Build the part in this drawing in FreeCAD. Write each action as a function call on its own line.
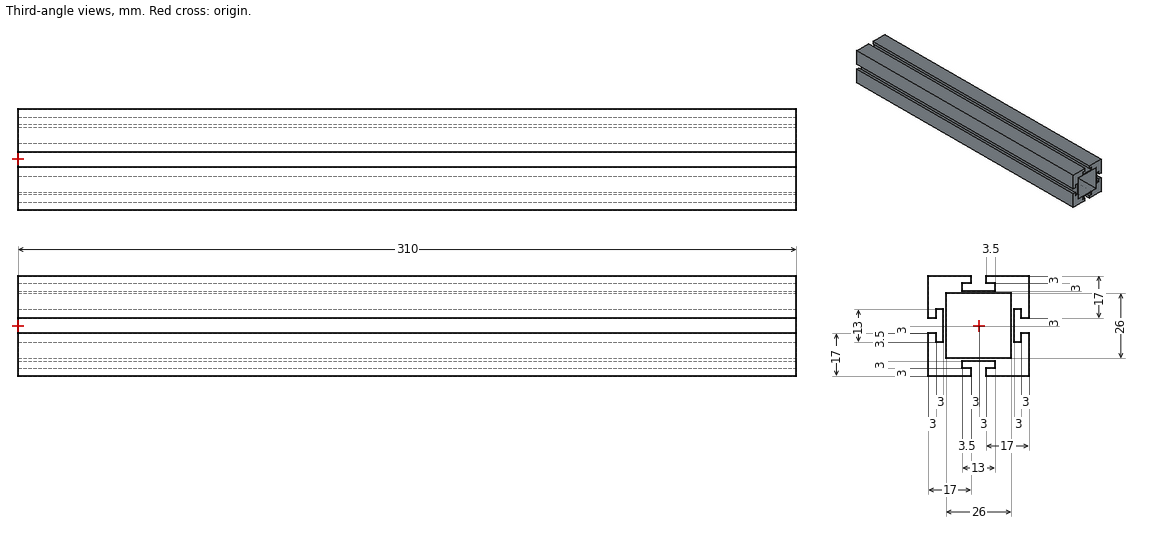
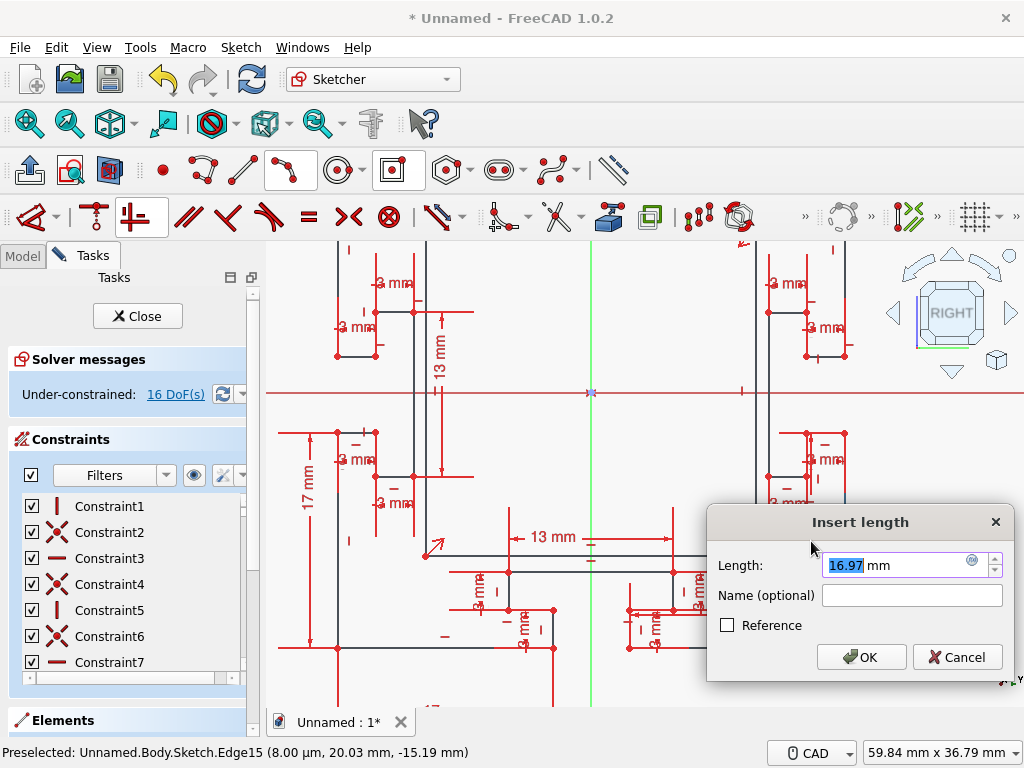
text(17)
key(Return)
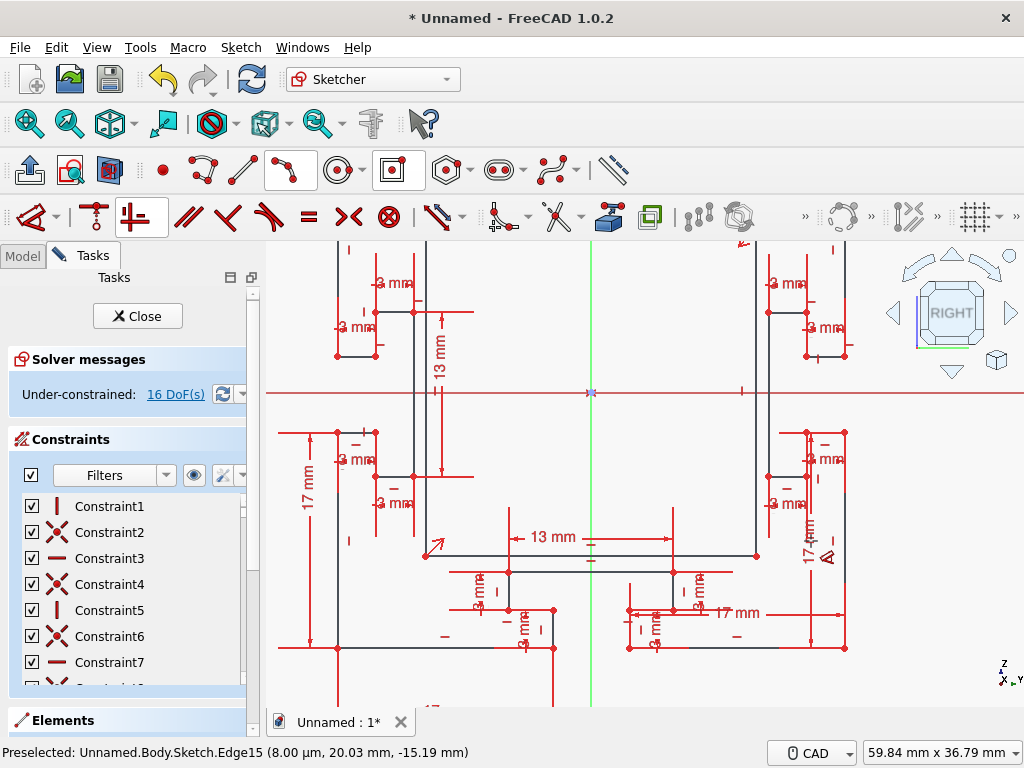
click(769, 428)
click(735, 357)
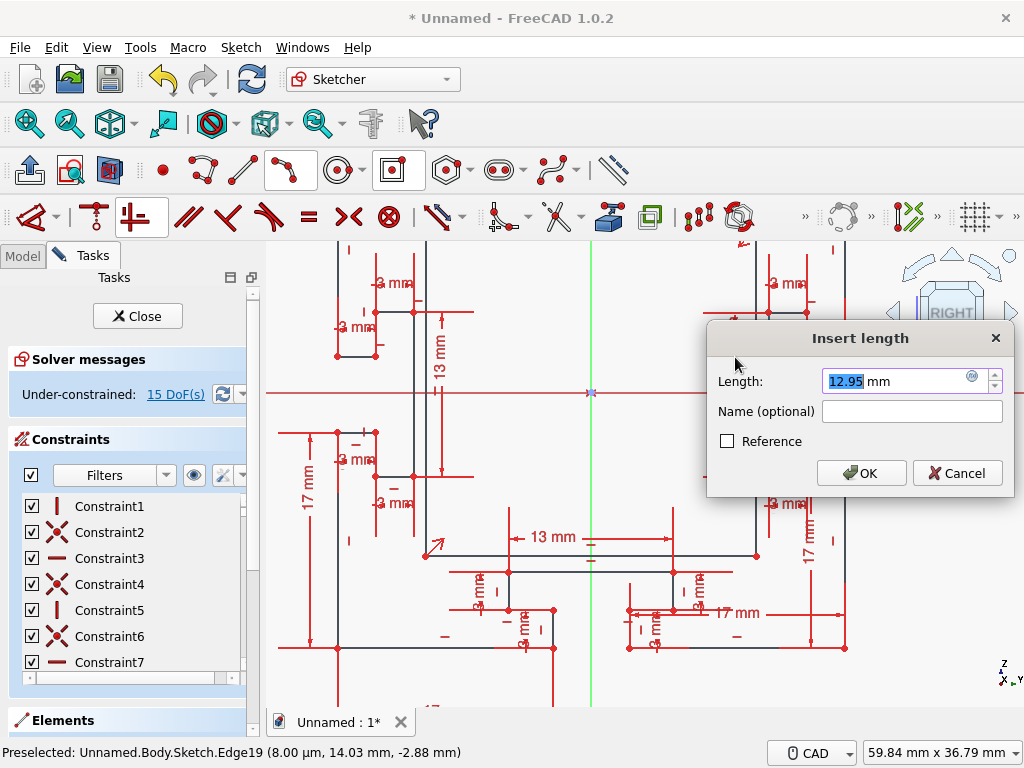
text(13)
key(Return)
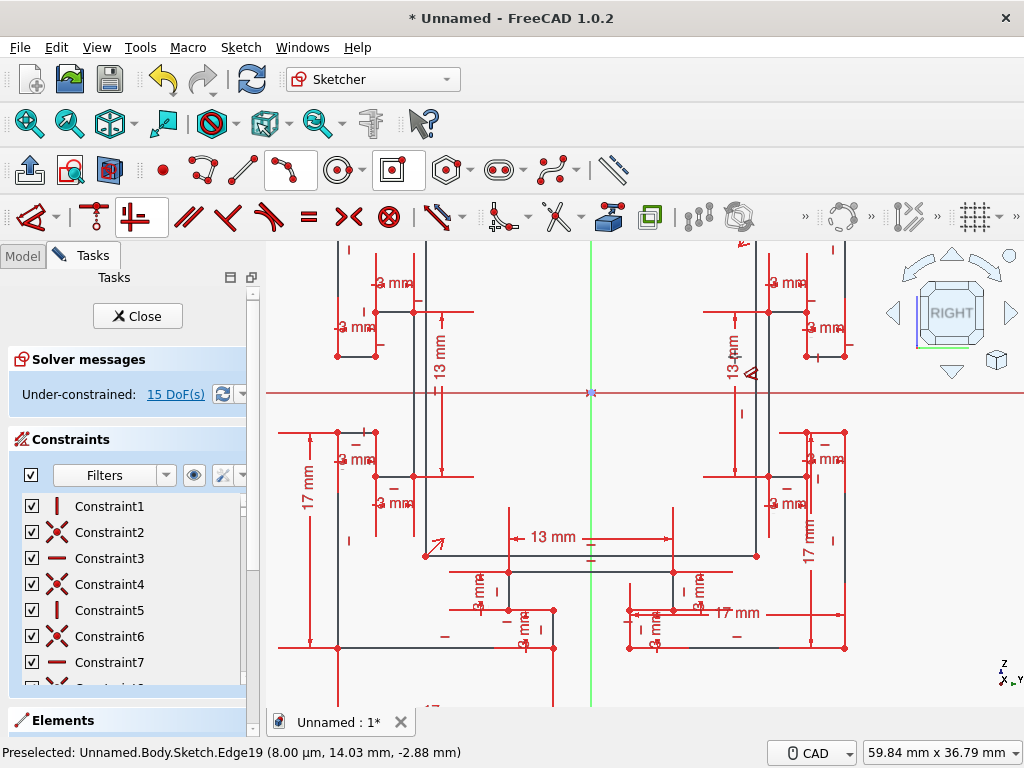
click(845, 292)
click(739, 313)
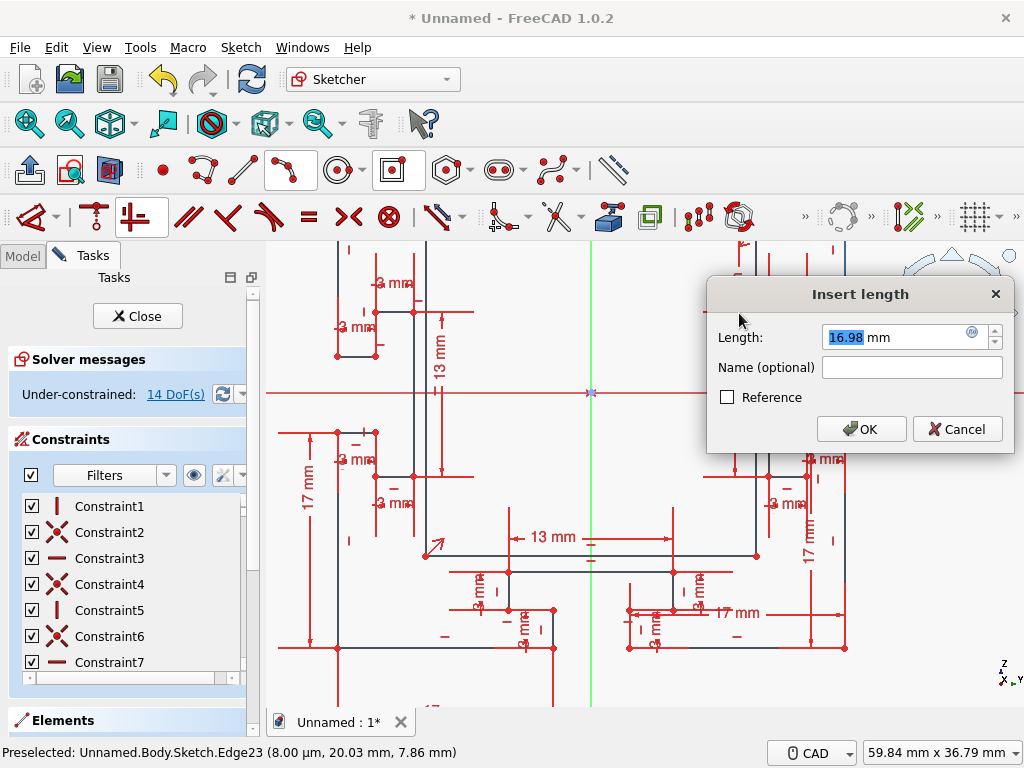
text(17)
key(Return)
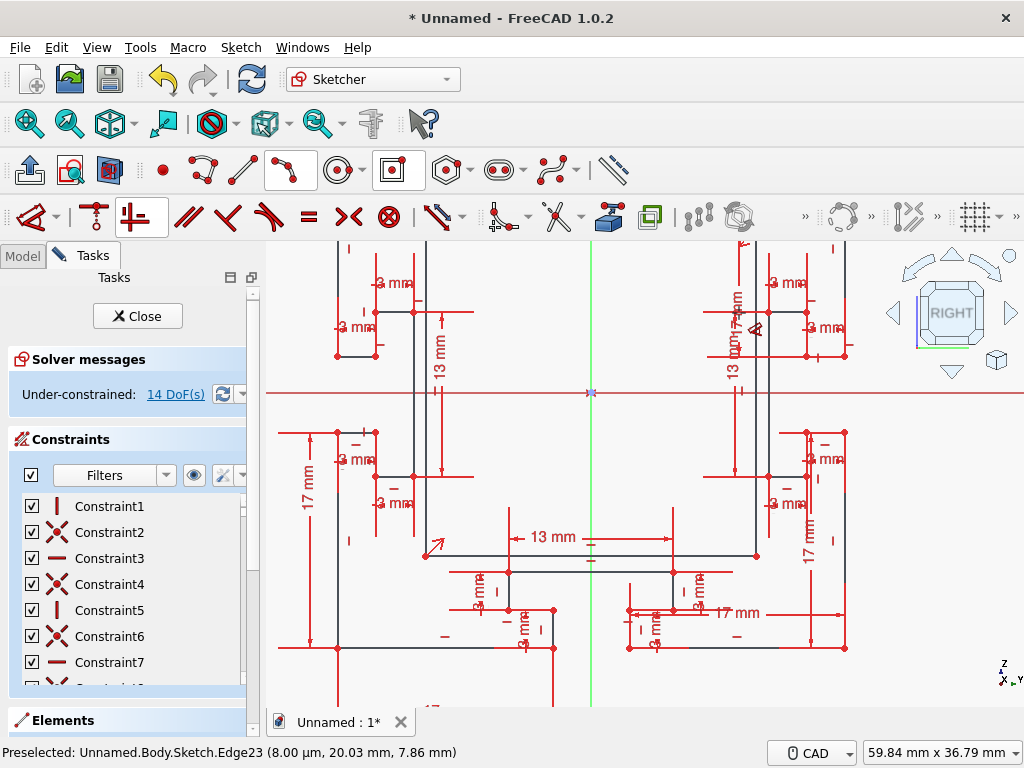
scroll(559, 573, down, 3)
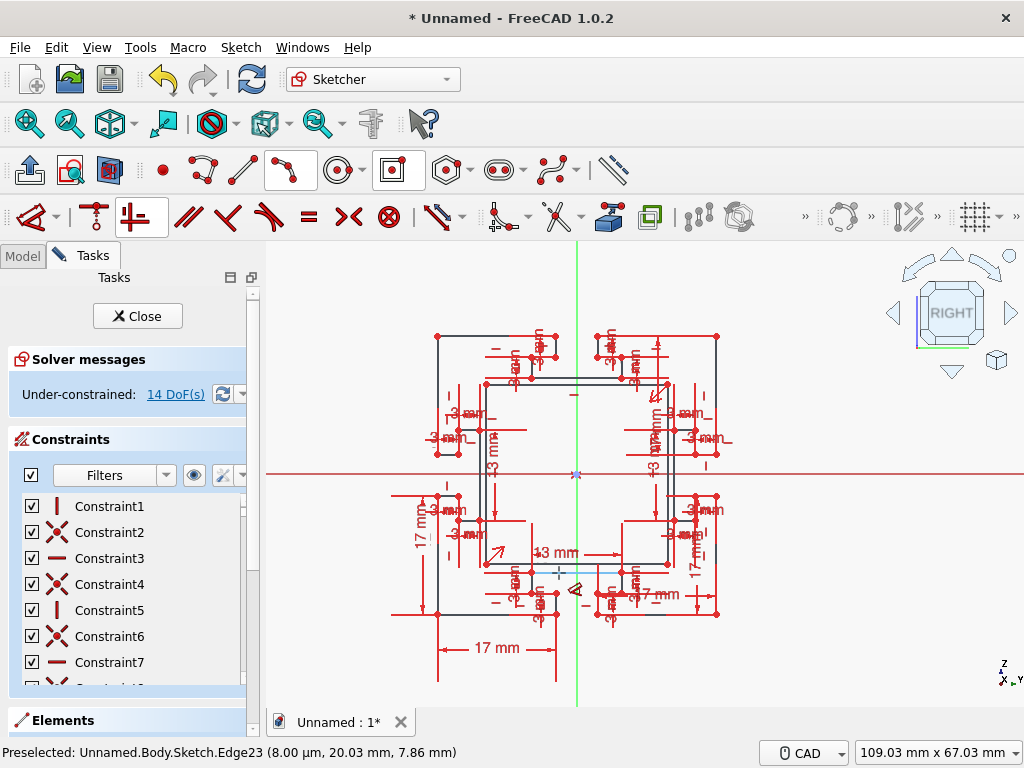
click(681, 336)
click(657, 302)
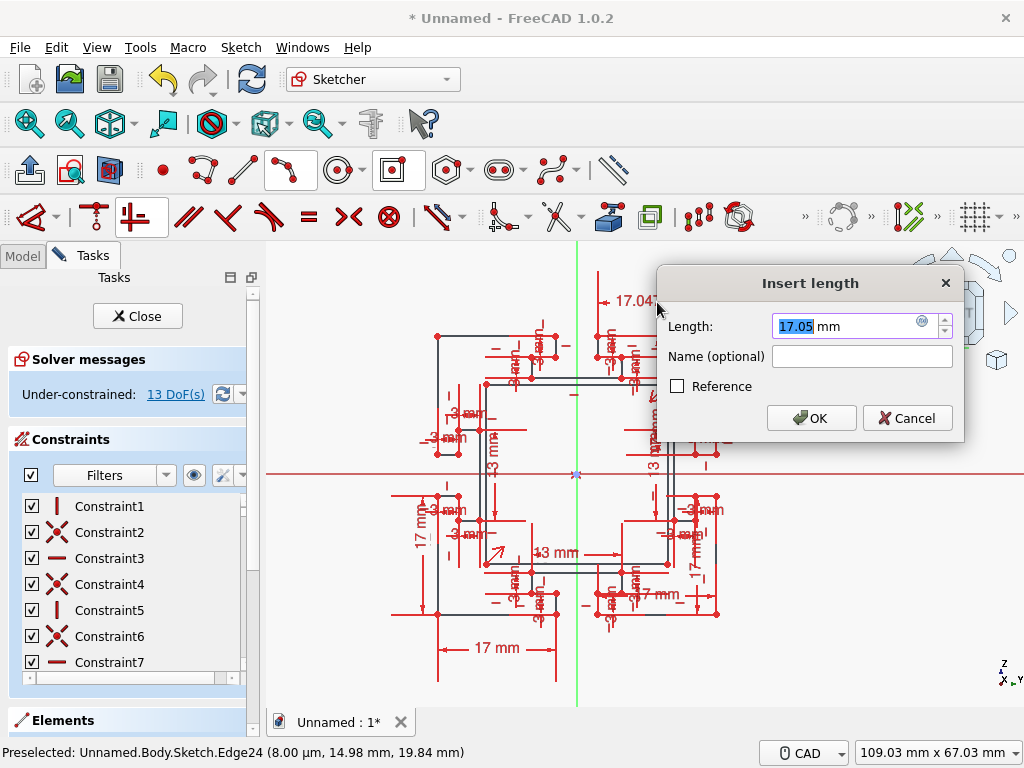
text(17)
key(Return)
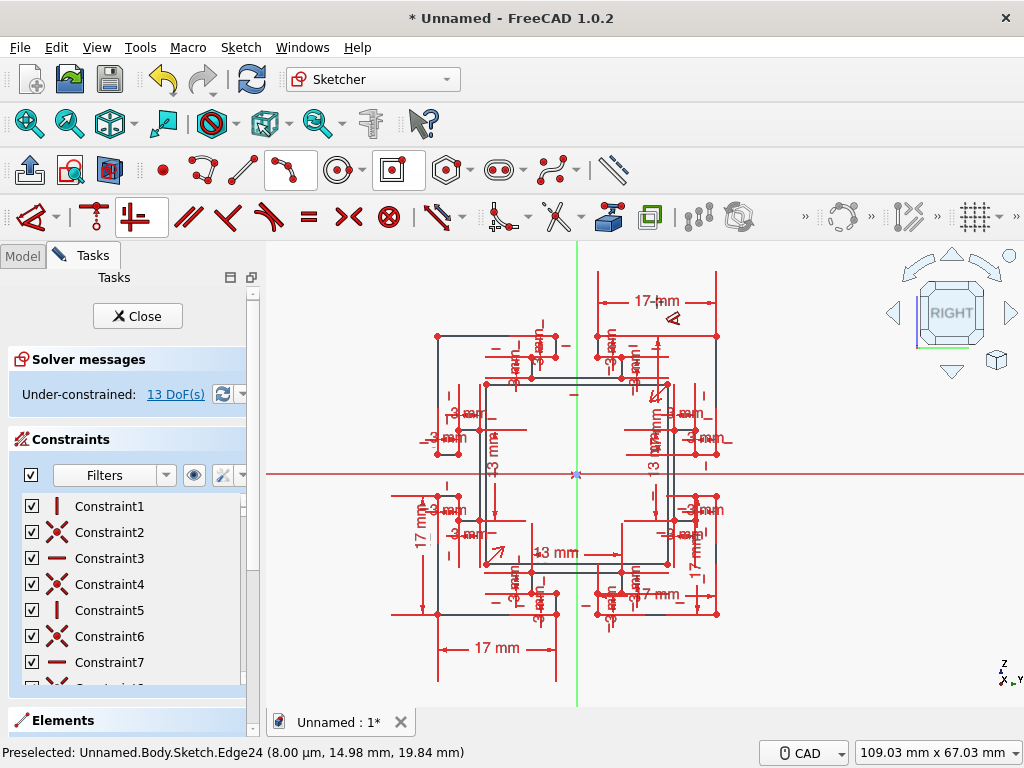
scroll(595, 378, up, 4)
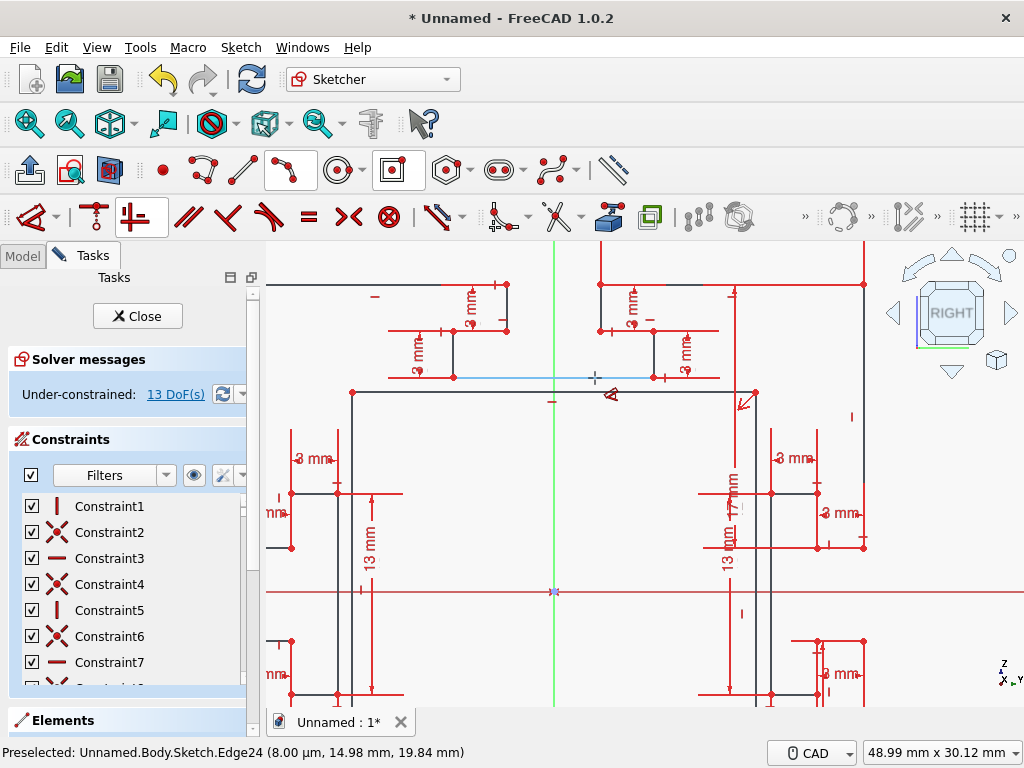
click(593, 378)
click(507, 412)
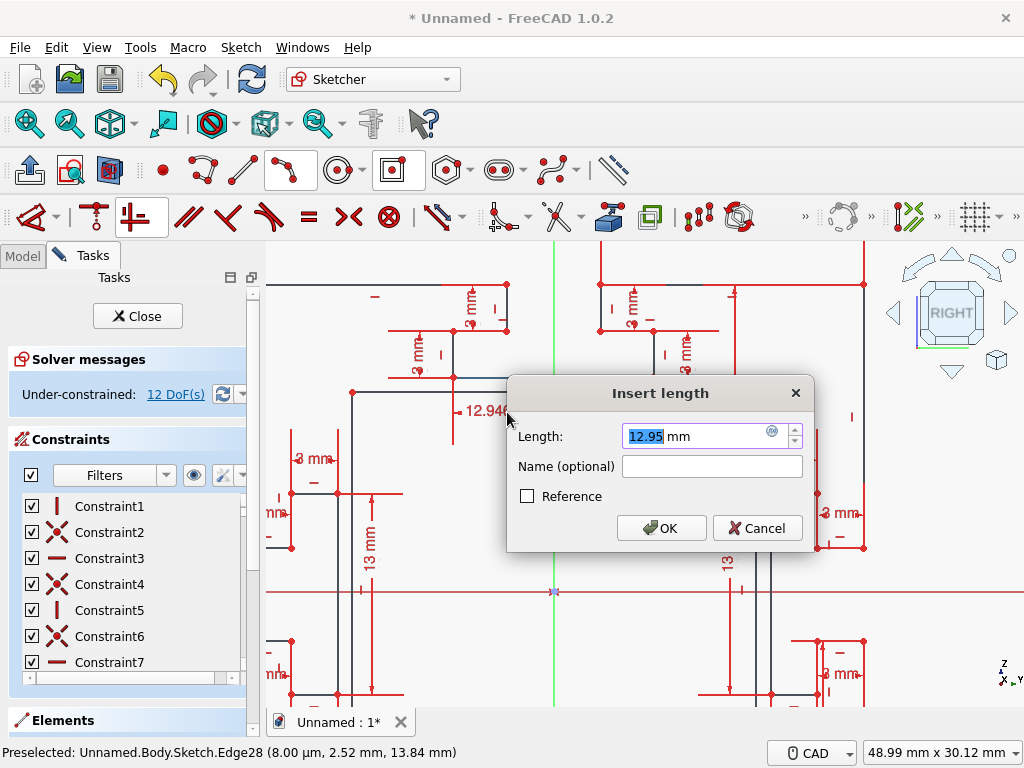
text(13)
key(Return)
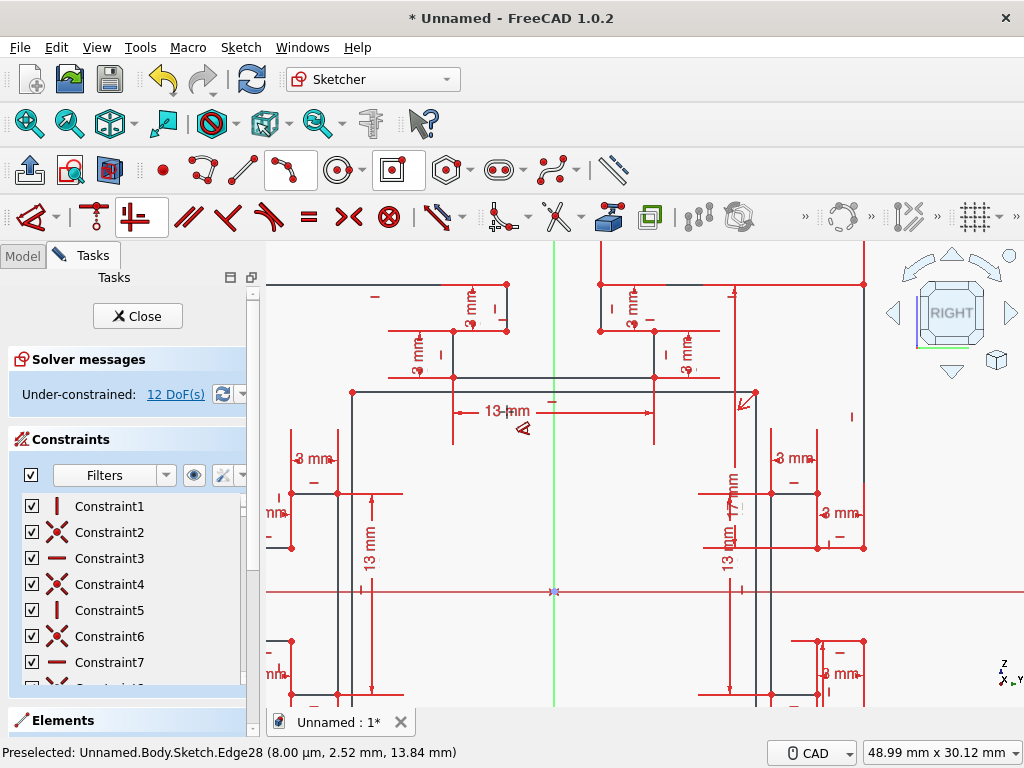
click(428, 285)
click(400, 319)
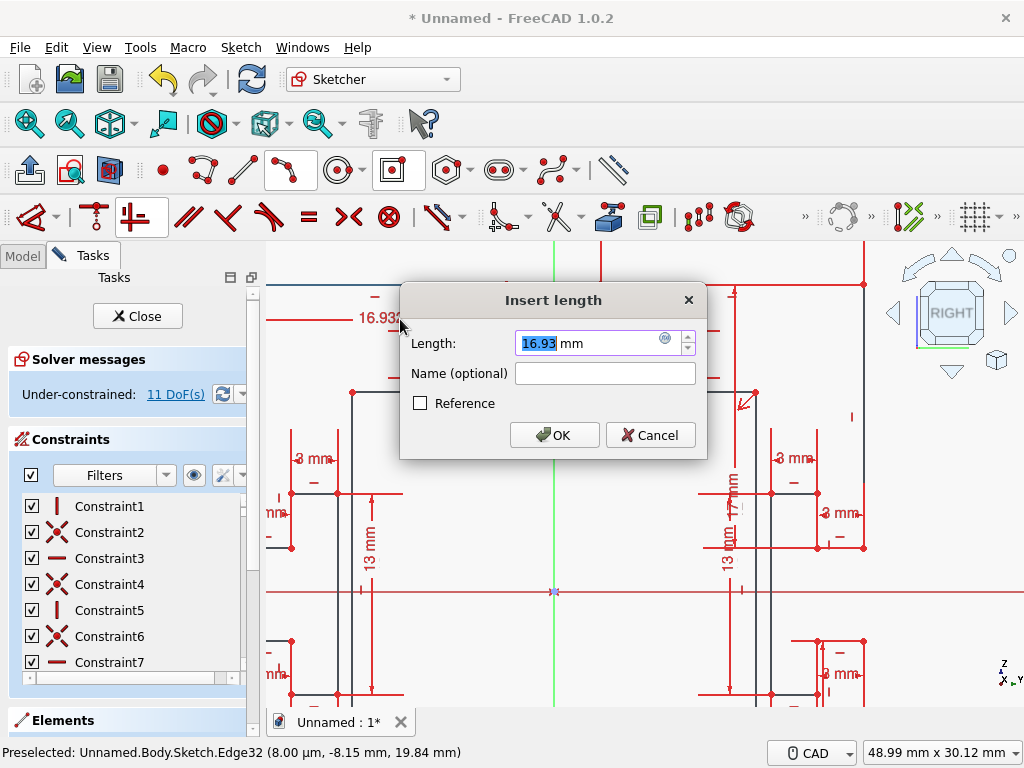
text(17)
key(Return)